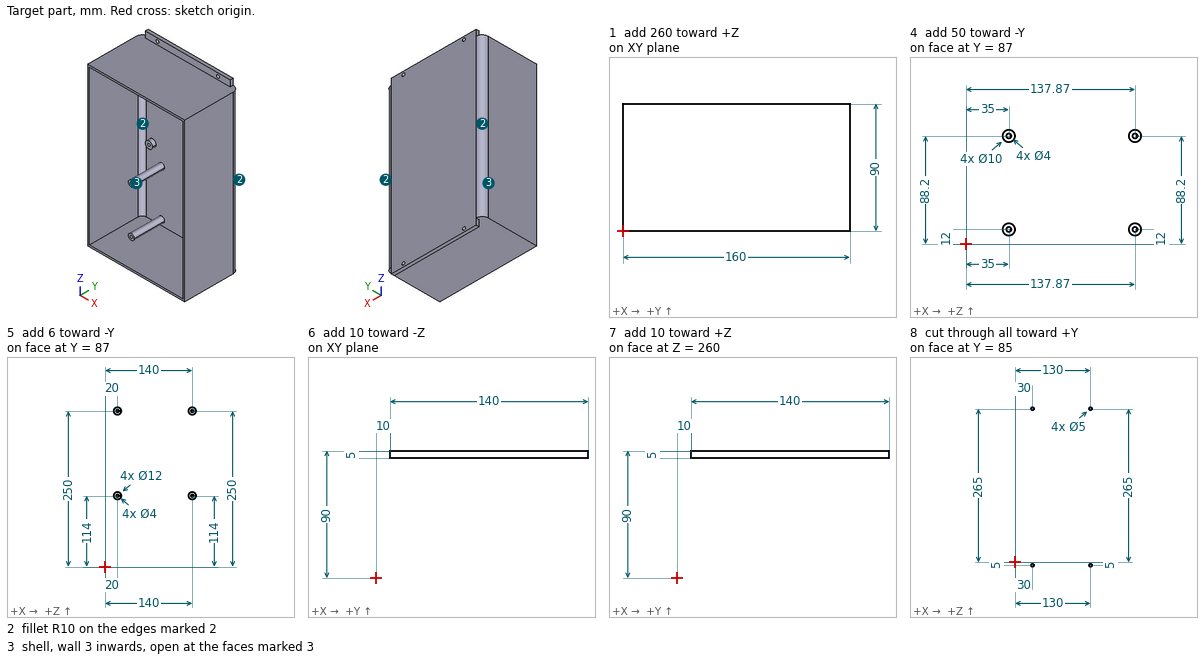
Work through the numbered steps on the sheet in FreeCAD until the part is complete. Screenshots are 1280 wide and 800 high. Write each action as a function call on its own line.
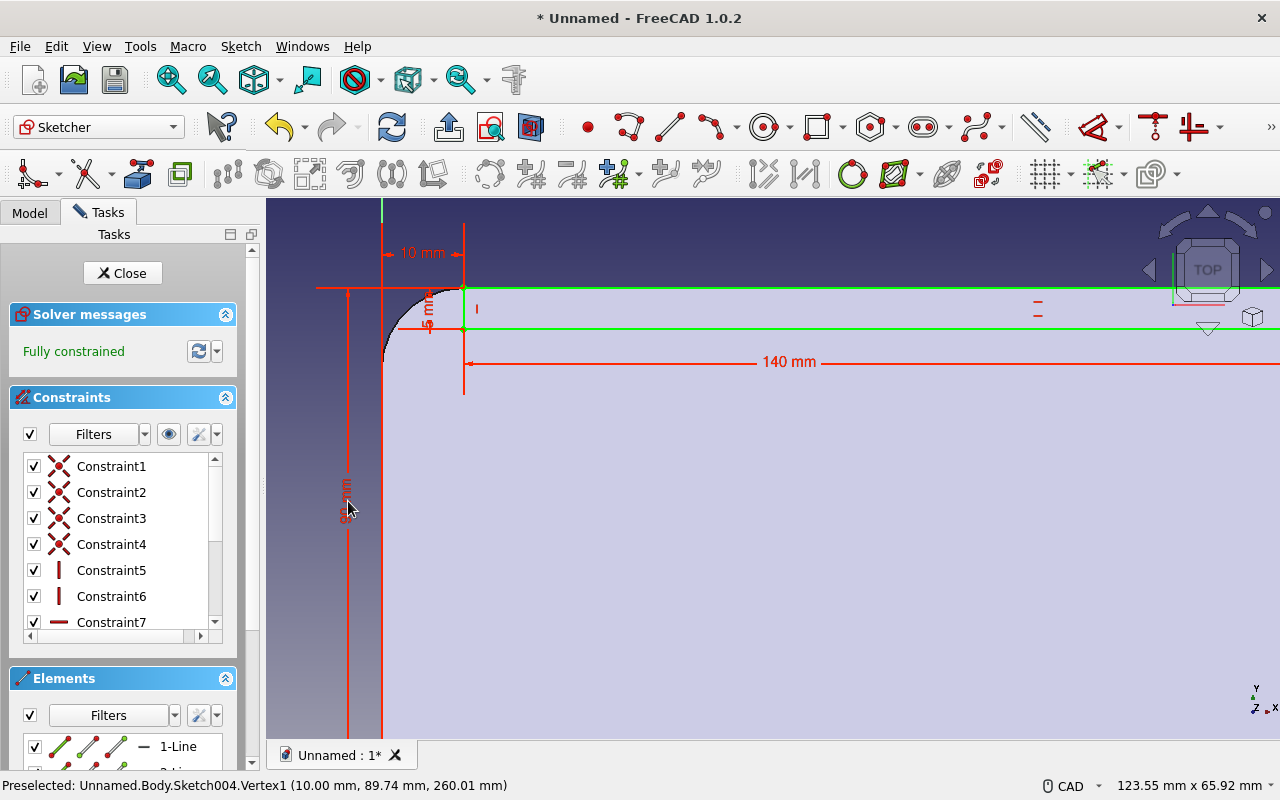
click(123, 273)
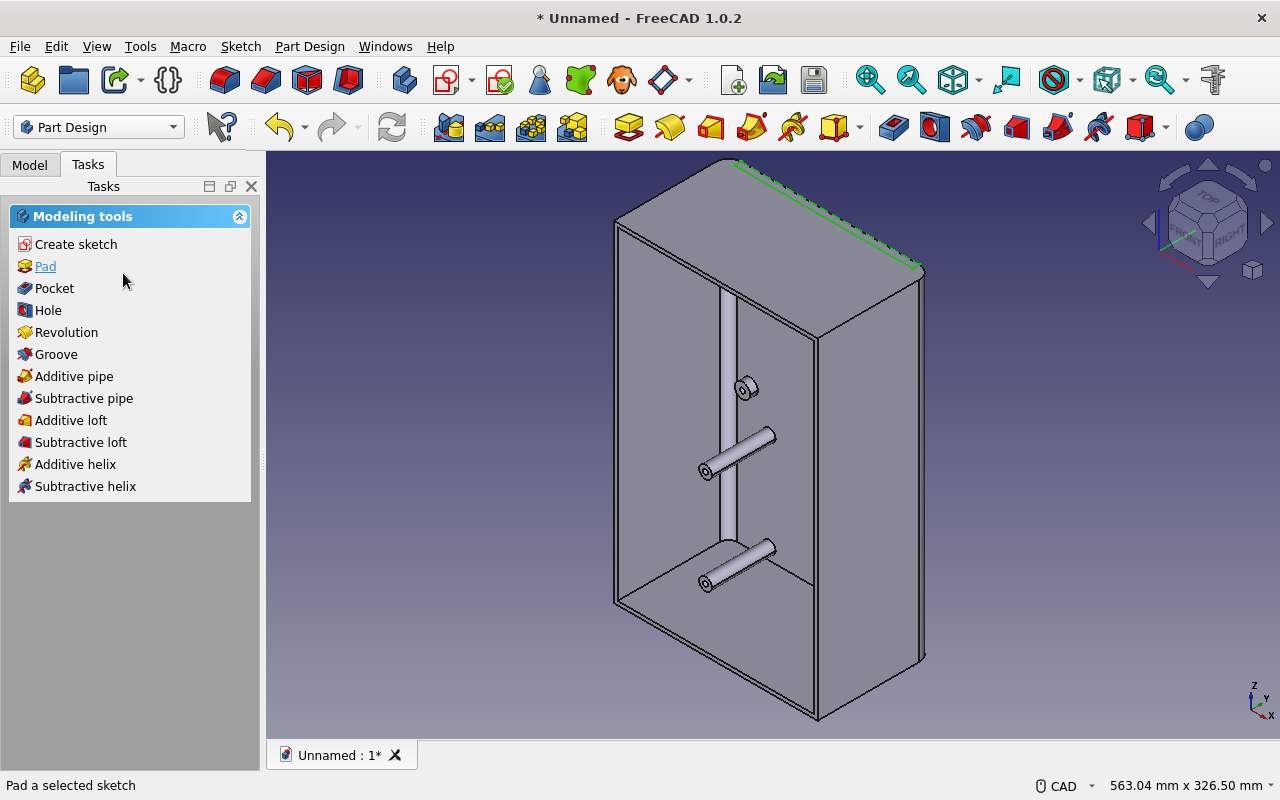
click(629, 128)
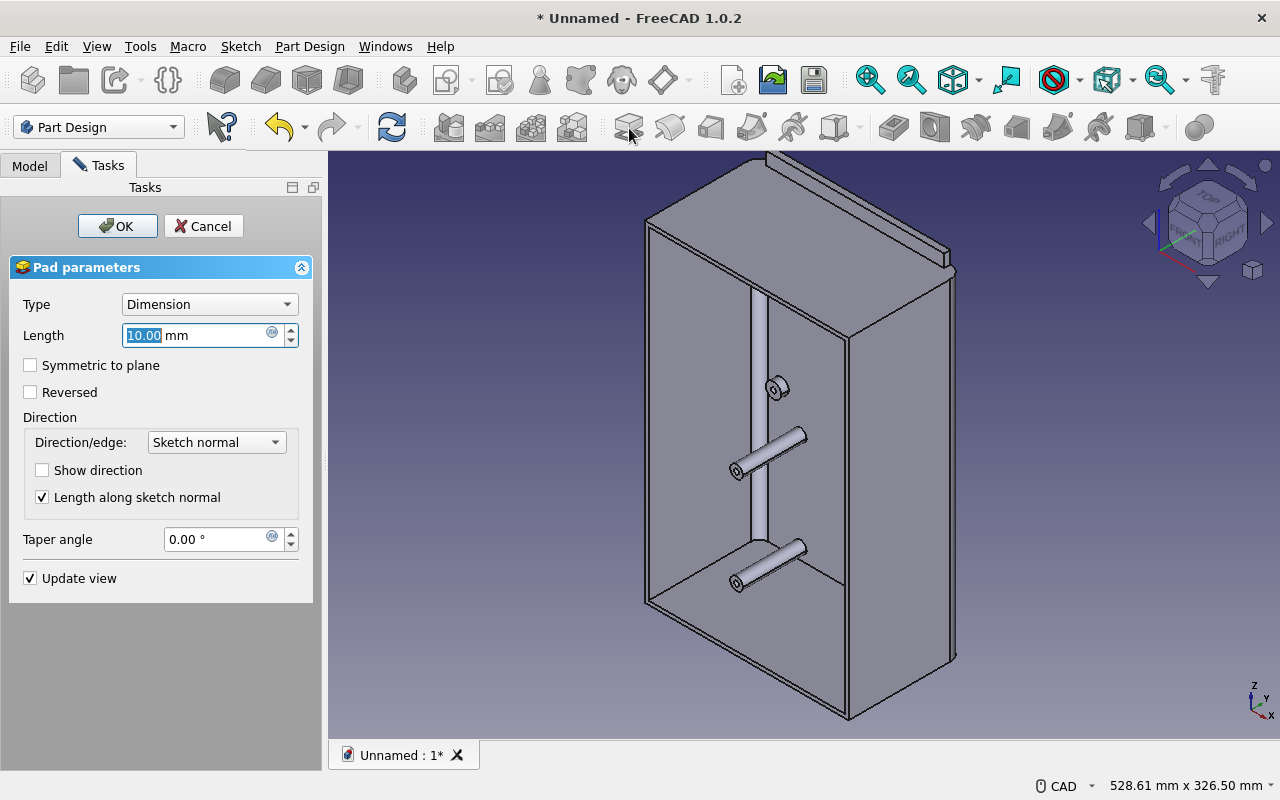
text(10)
key(Tab)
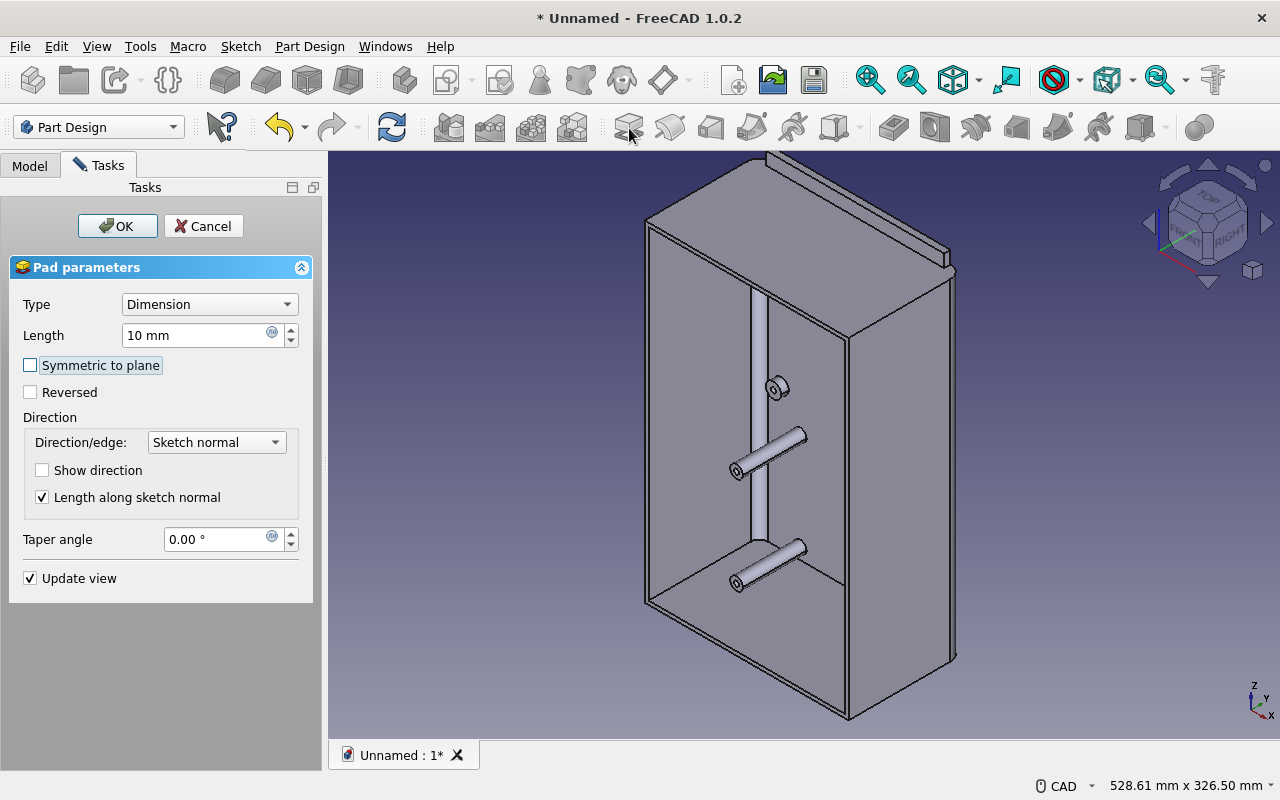
click(118, 226)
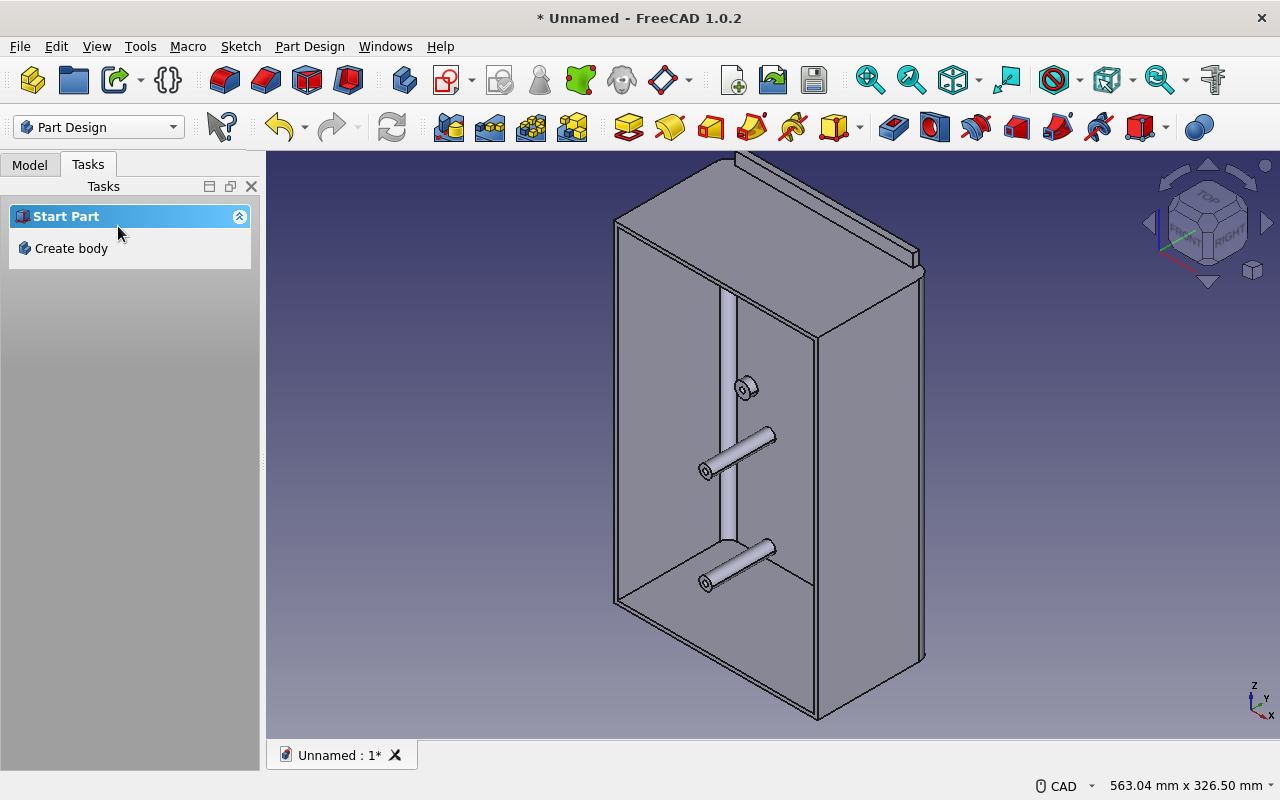
click(871, 80)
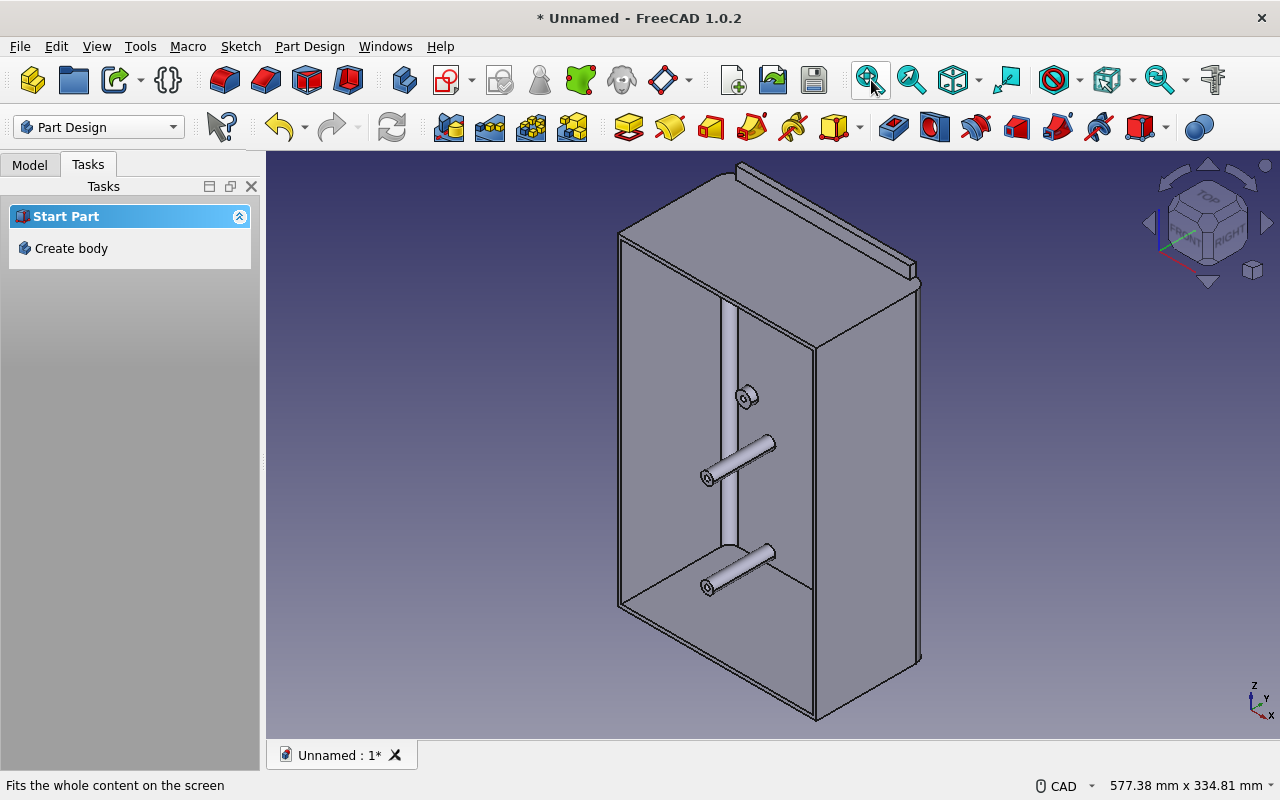
key(1)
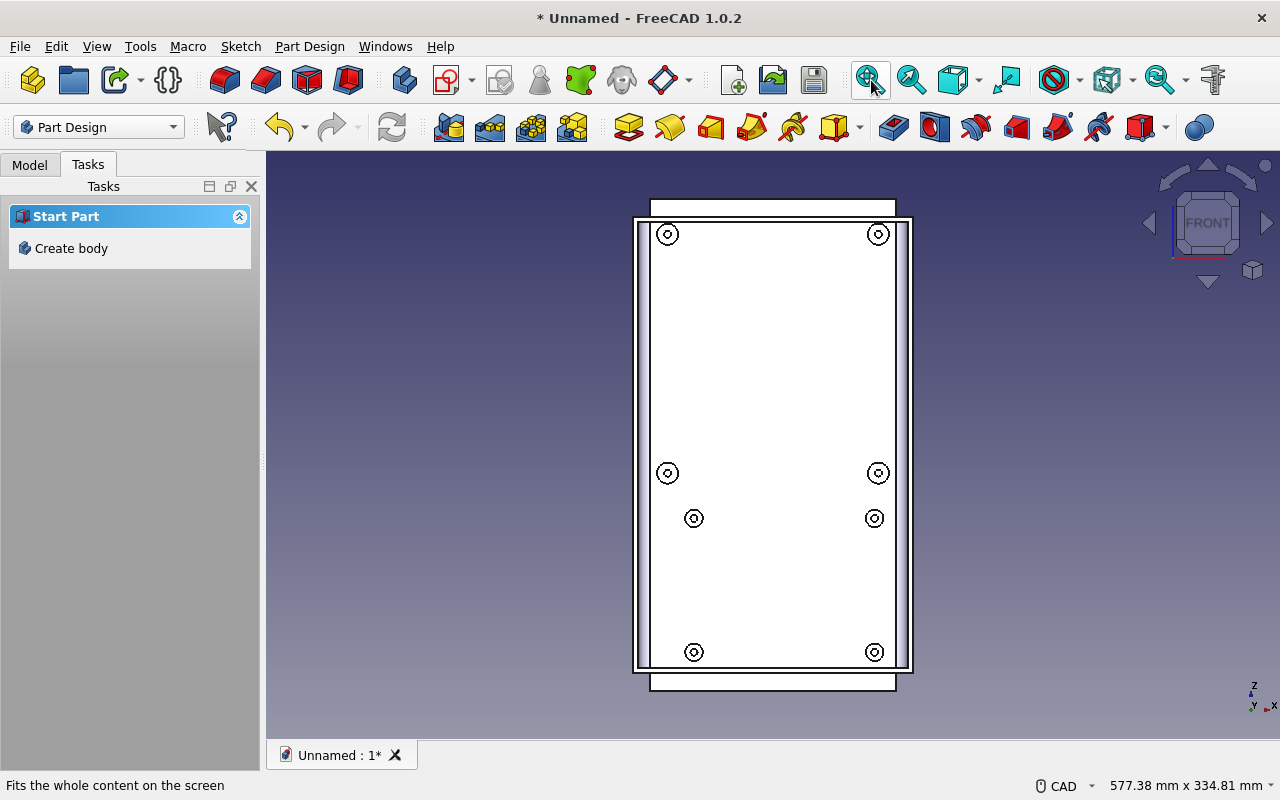
click(878, 681)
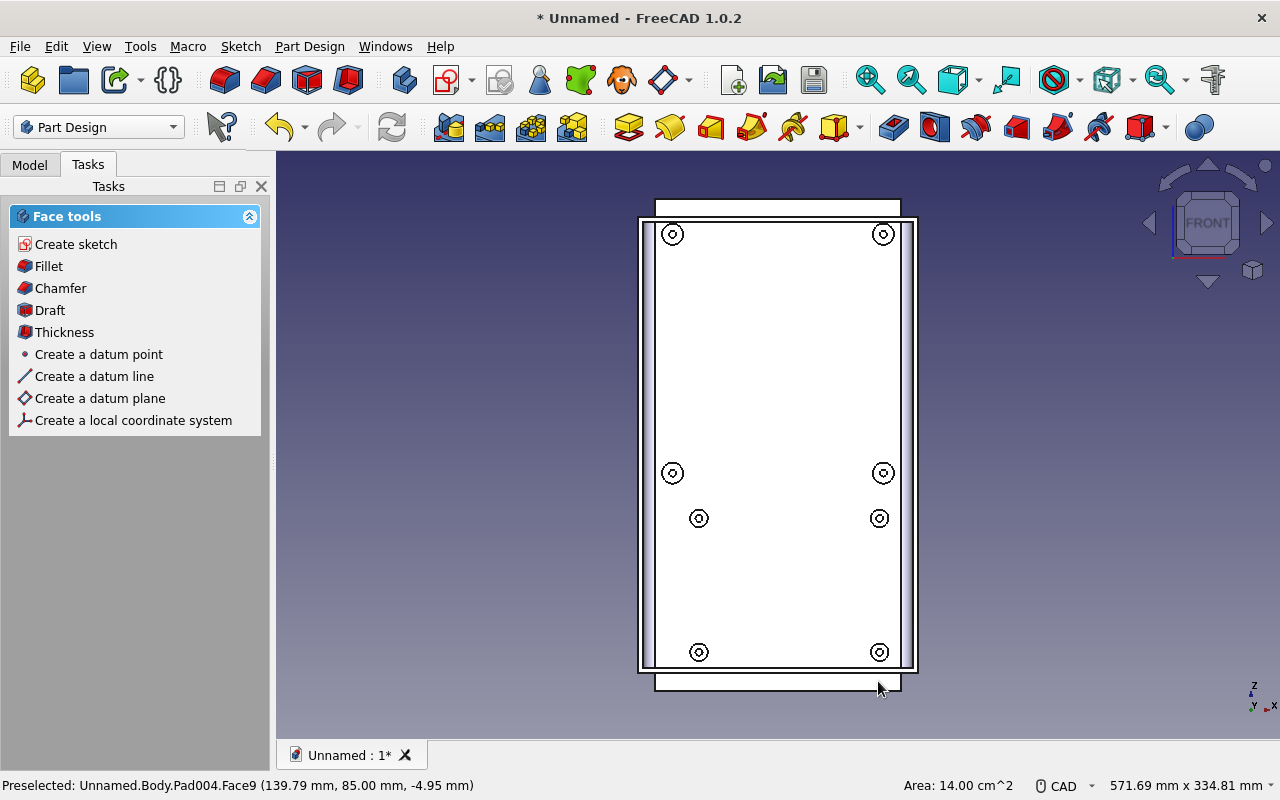
click(446, 80)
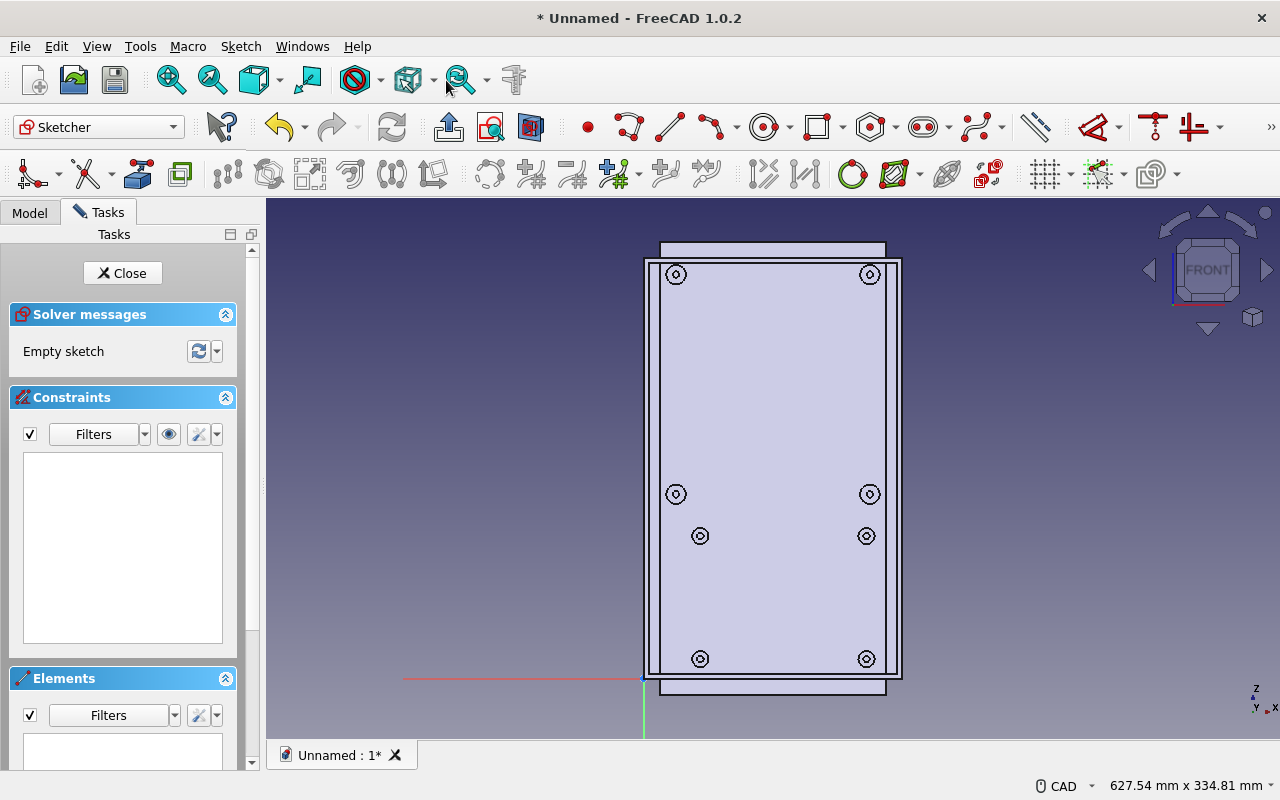
scroll(495, 469, down, 1)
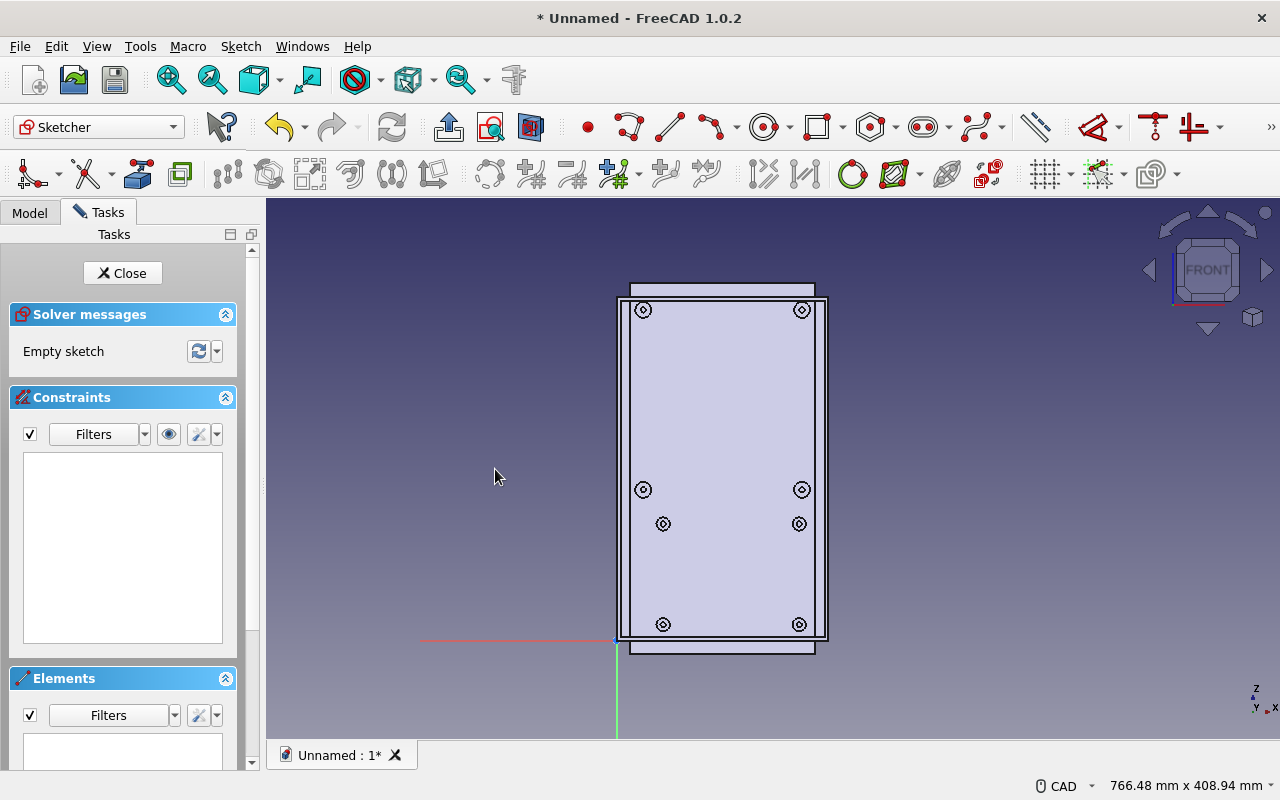
key(g)
key(c)